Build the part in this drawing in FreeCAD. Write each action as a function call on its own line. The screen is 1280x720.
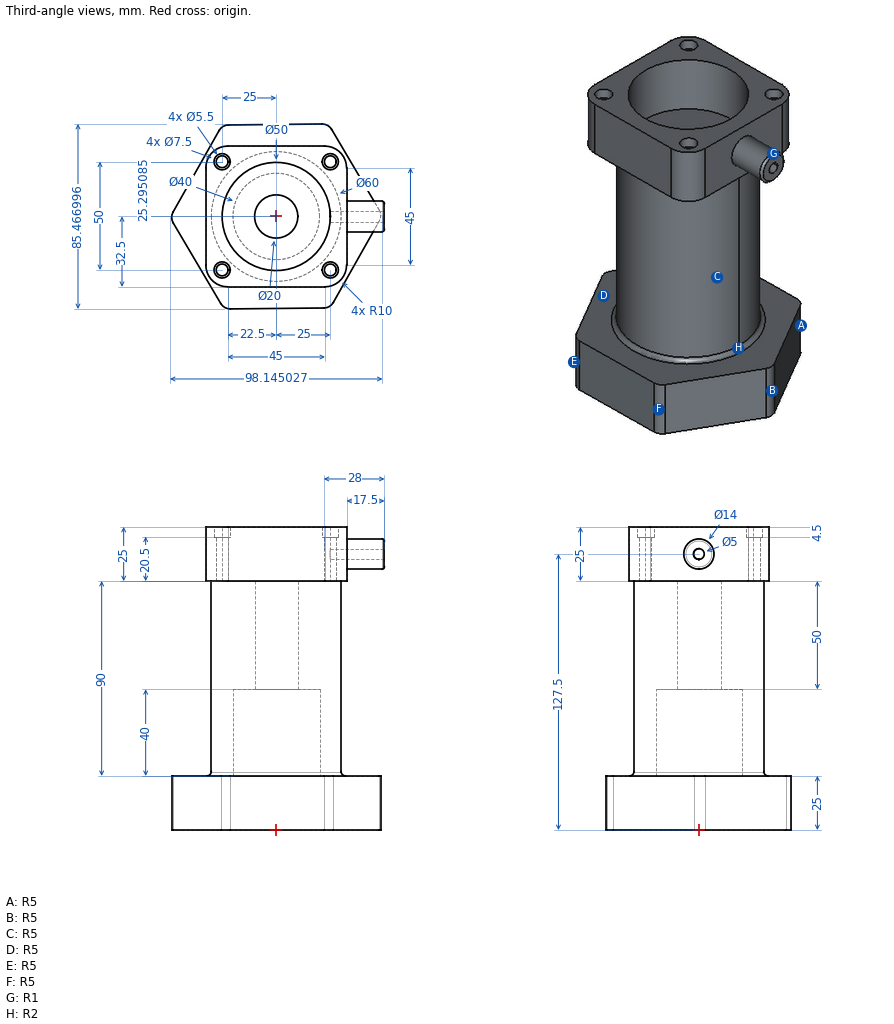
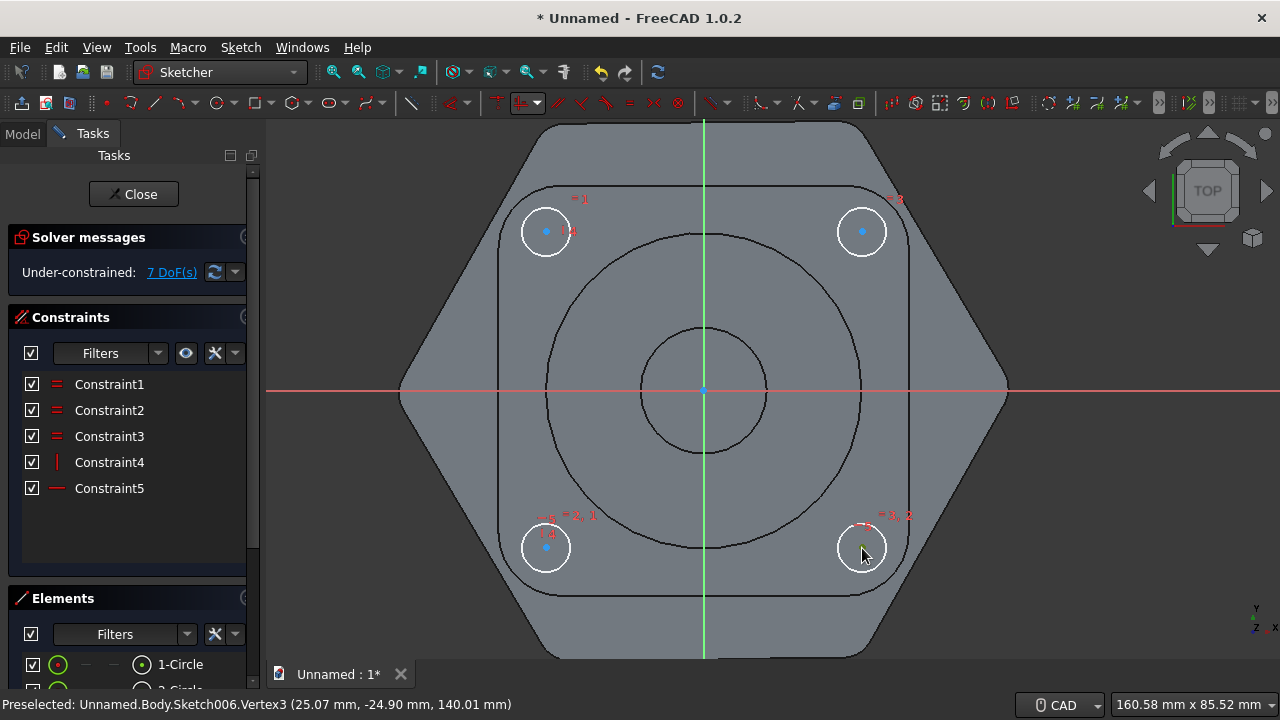
click(862, 232)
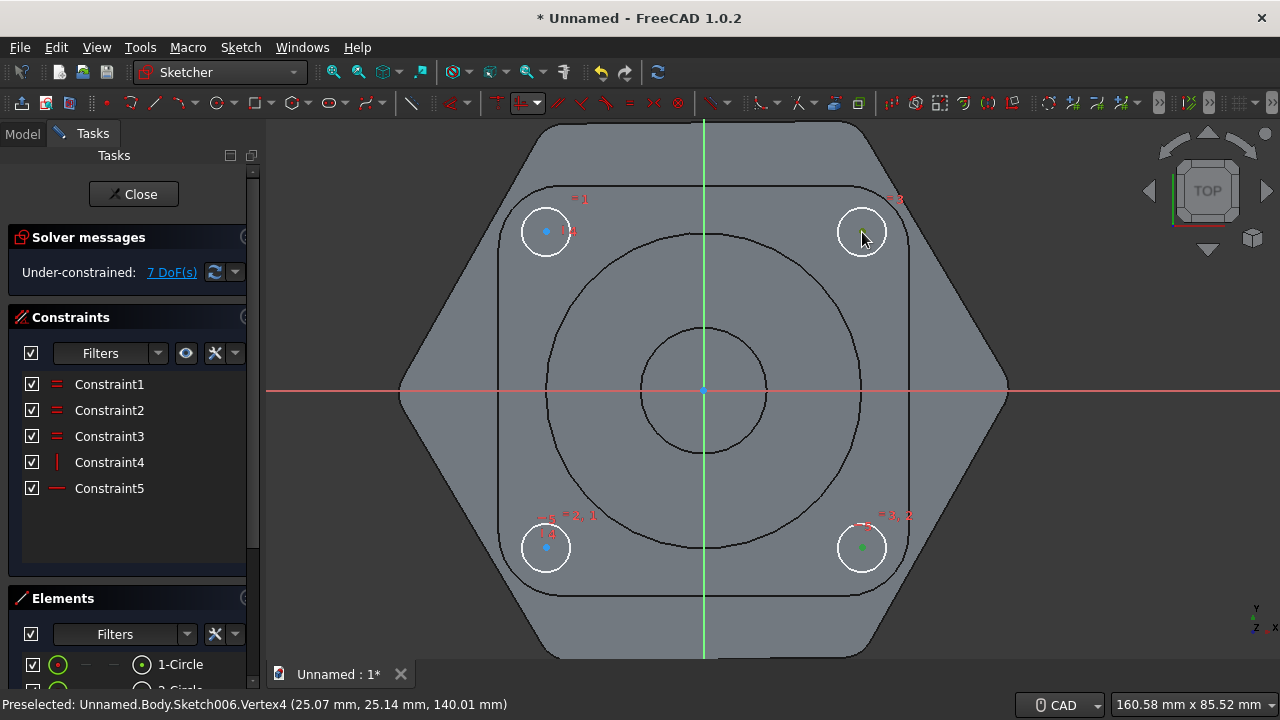
key(v)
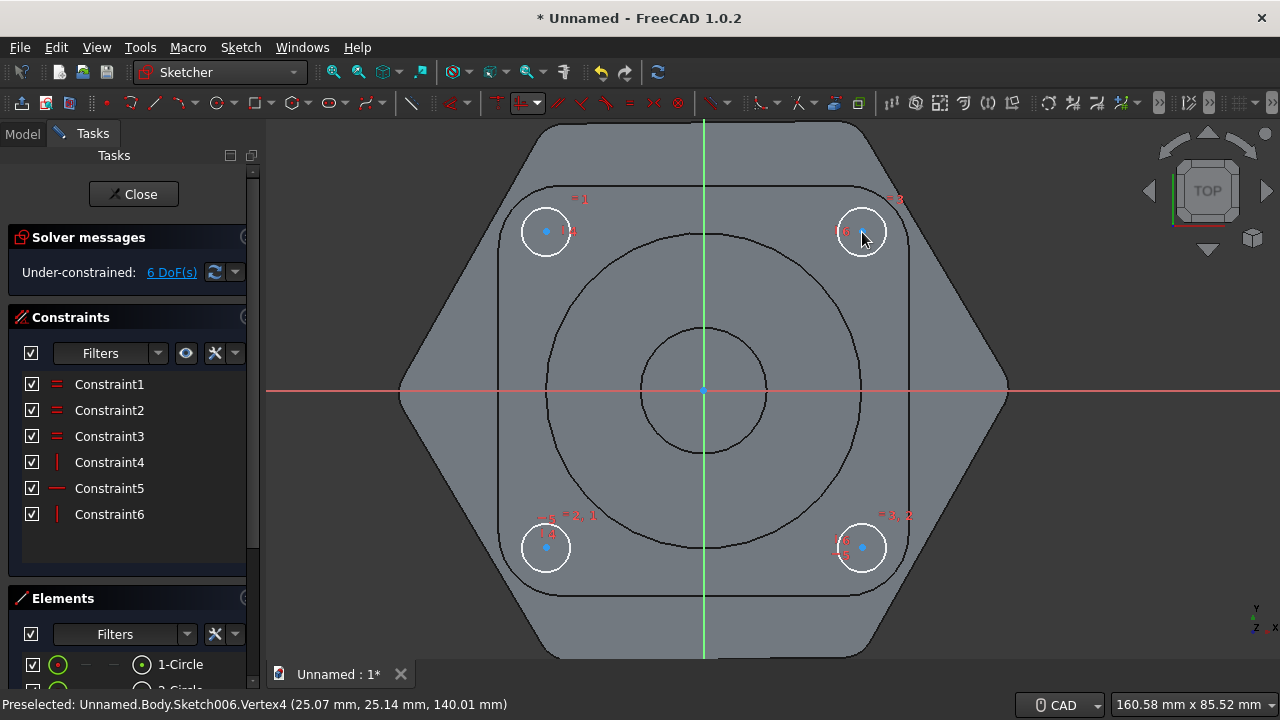
click(546, 232)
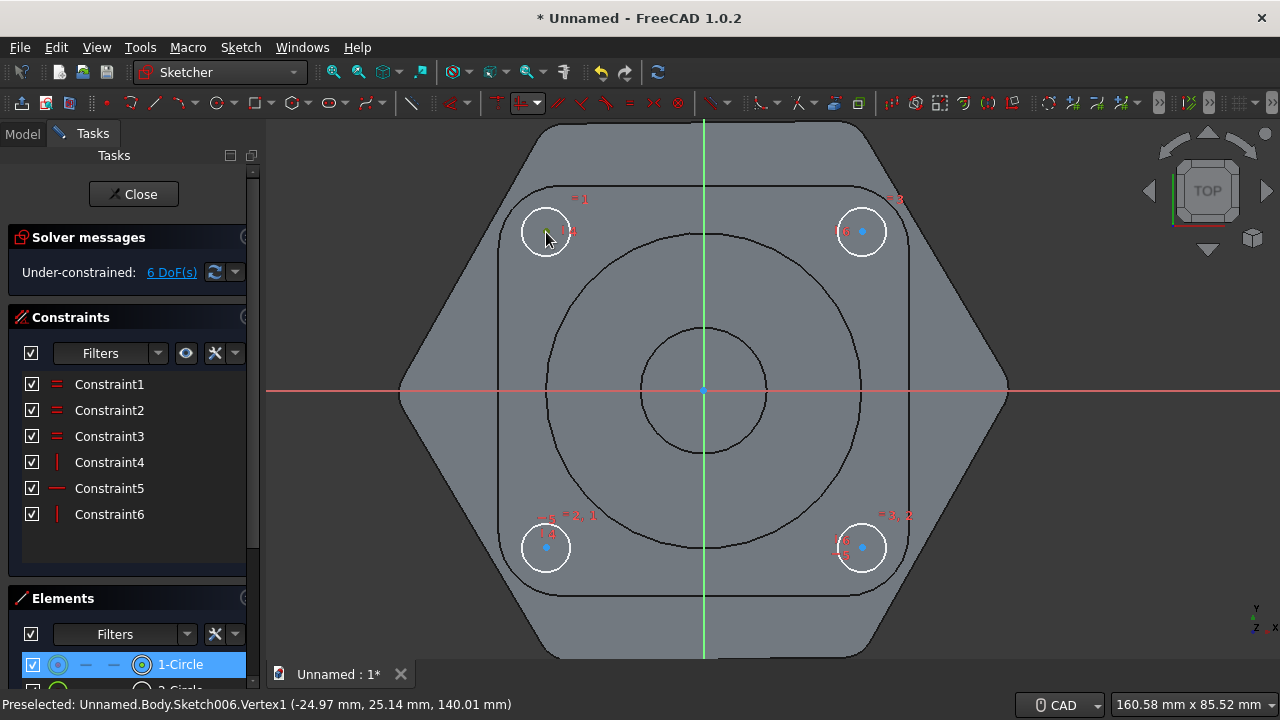
click(862, 232)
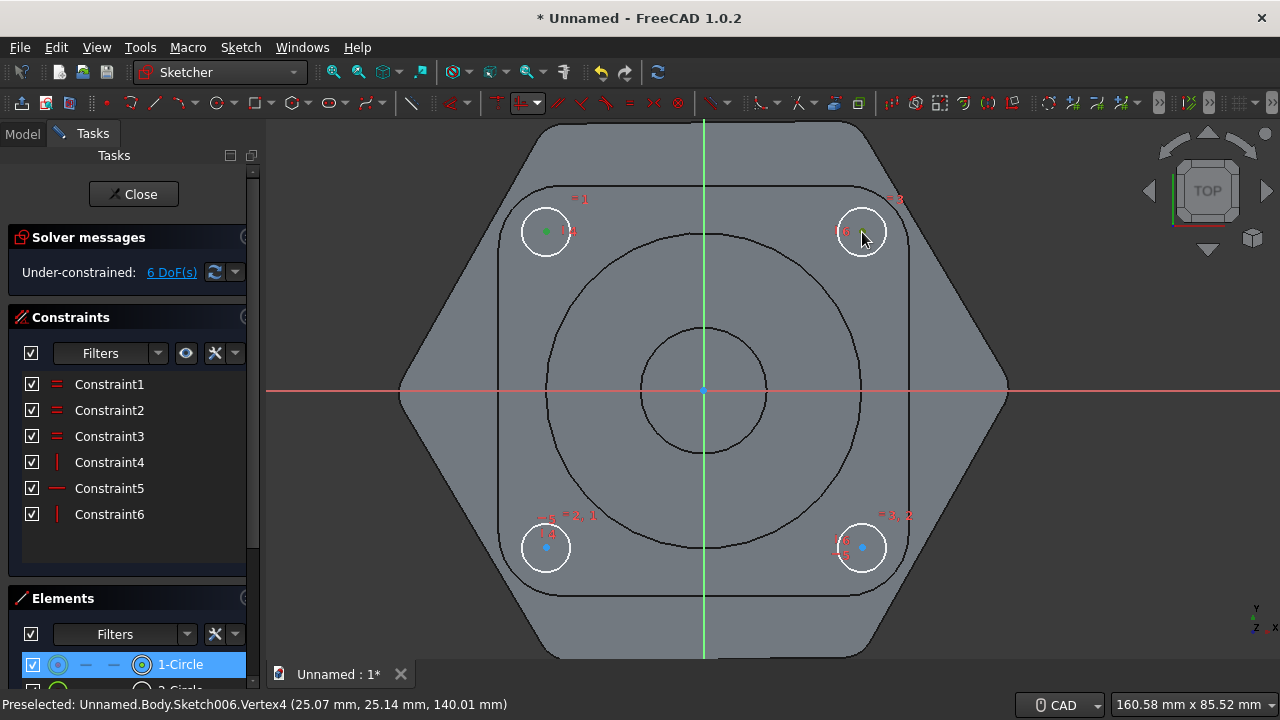
click(540, 104)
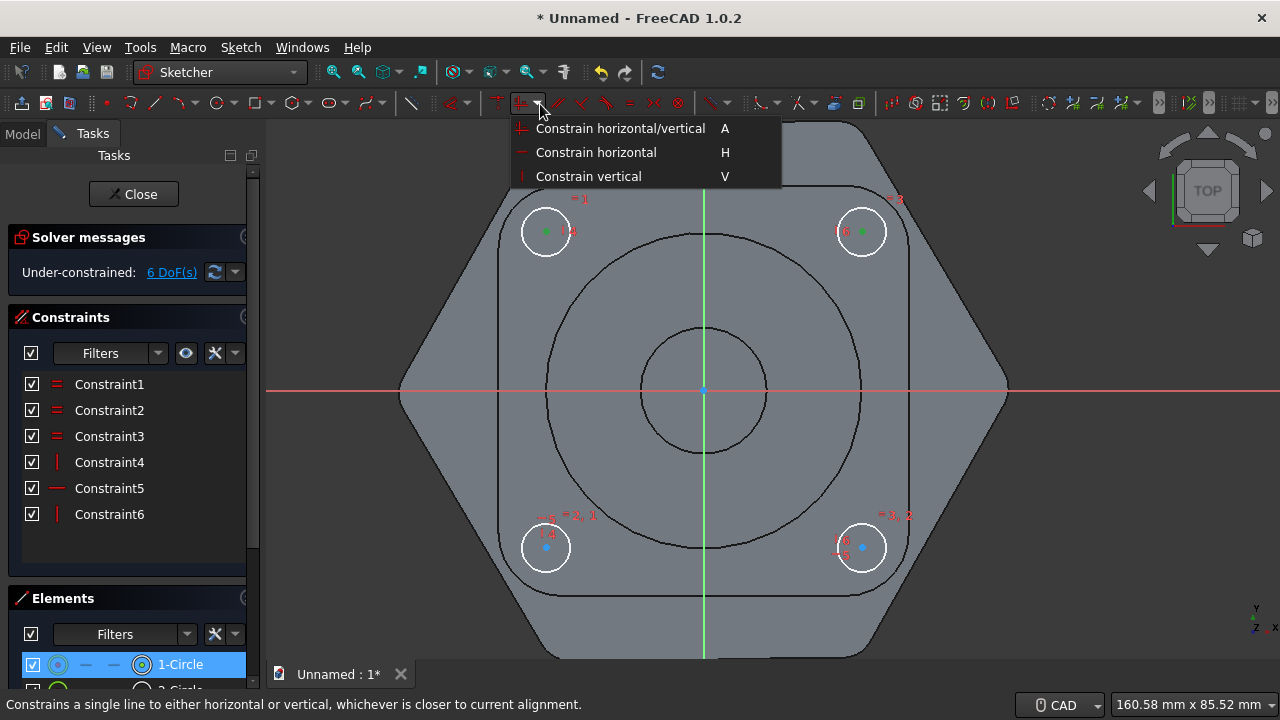
click(646, 152)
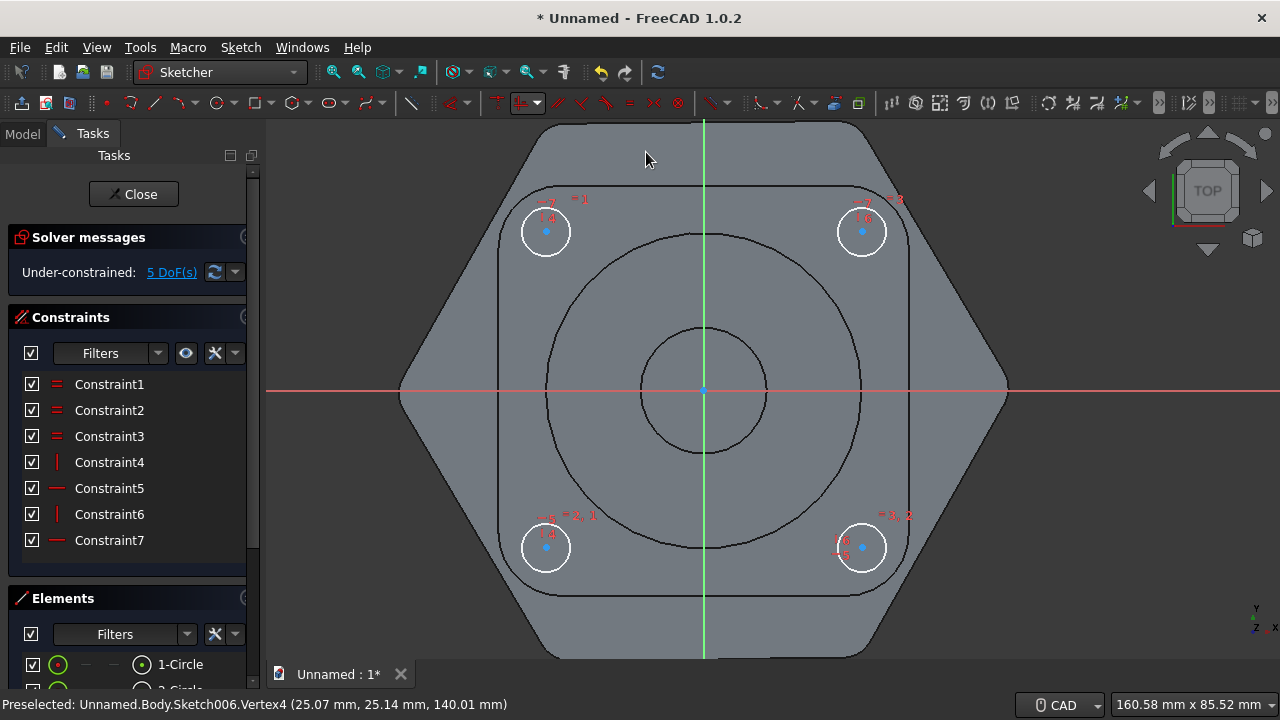
click(450, 104)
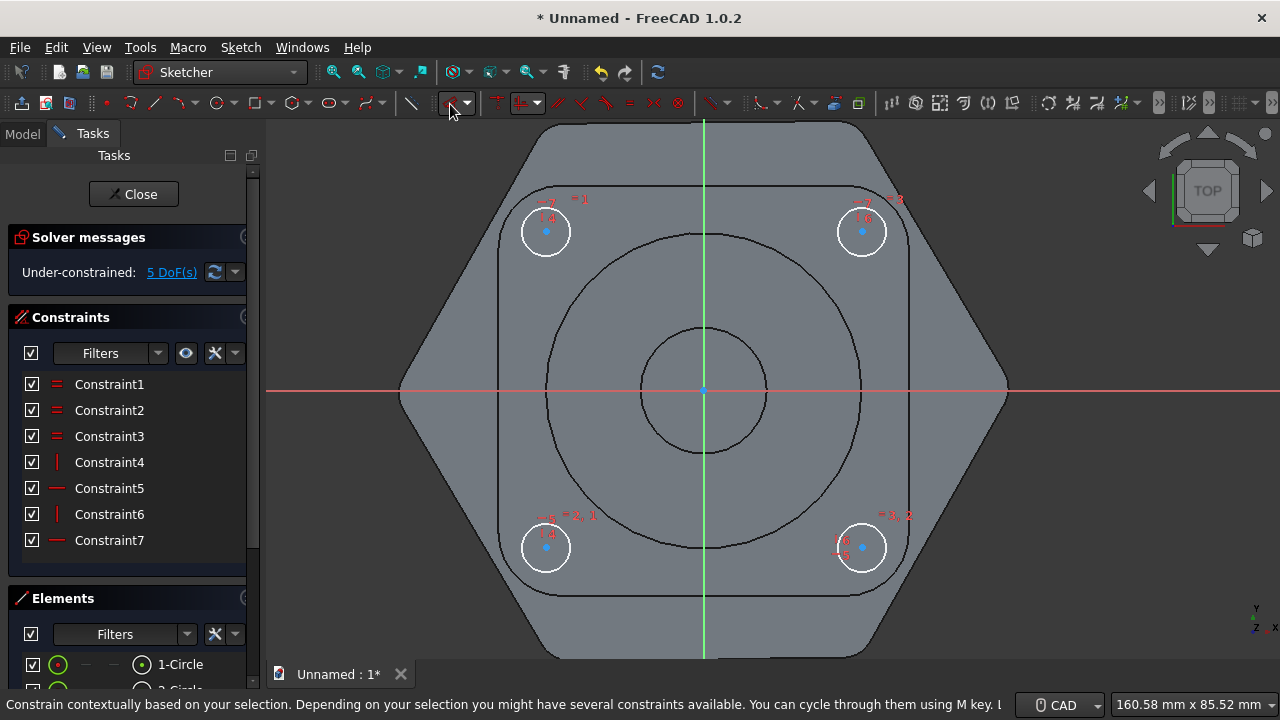
click(563, 215)
click(586, 192)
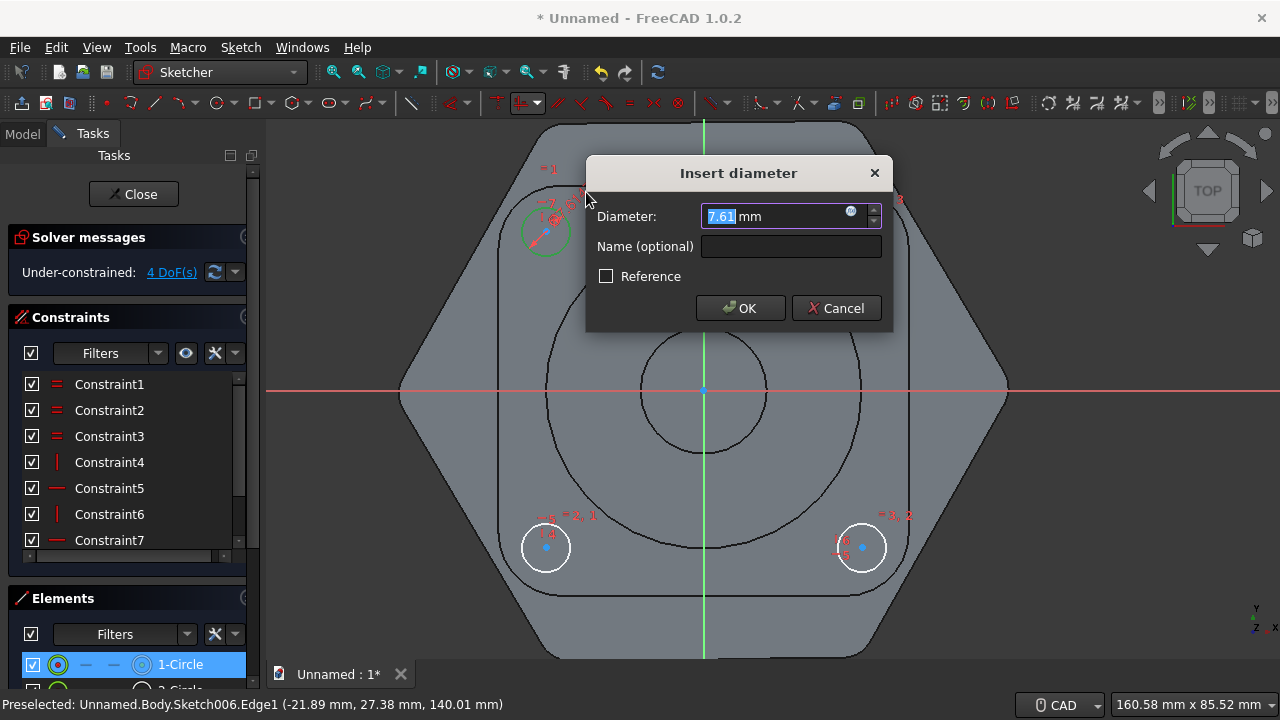
text(7.5)
key(Return)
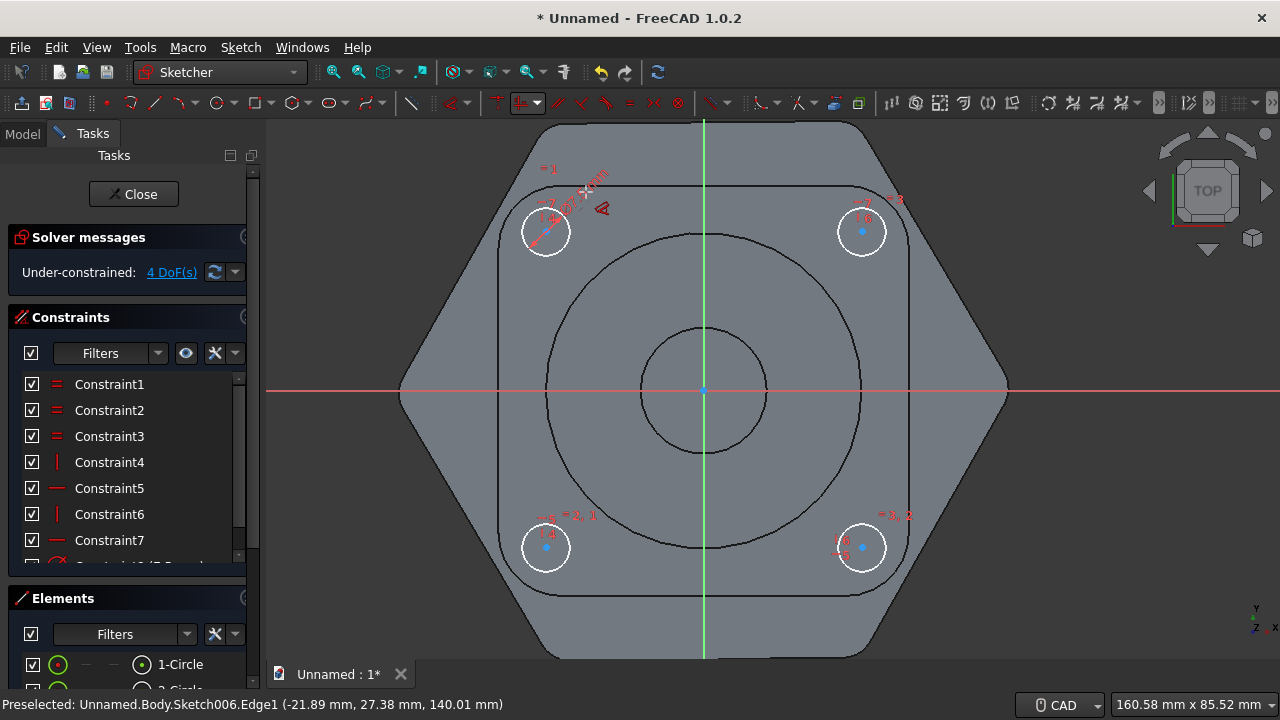
click(546, 232)
click(661, 198)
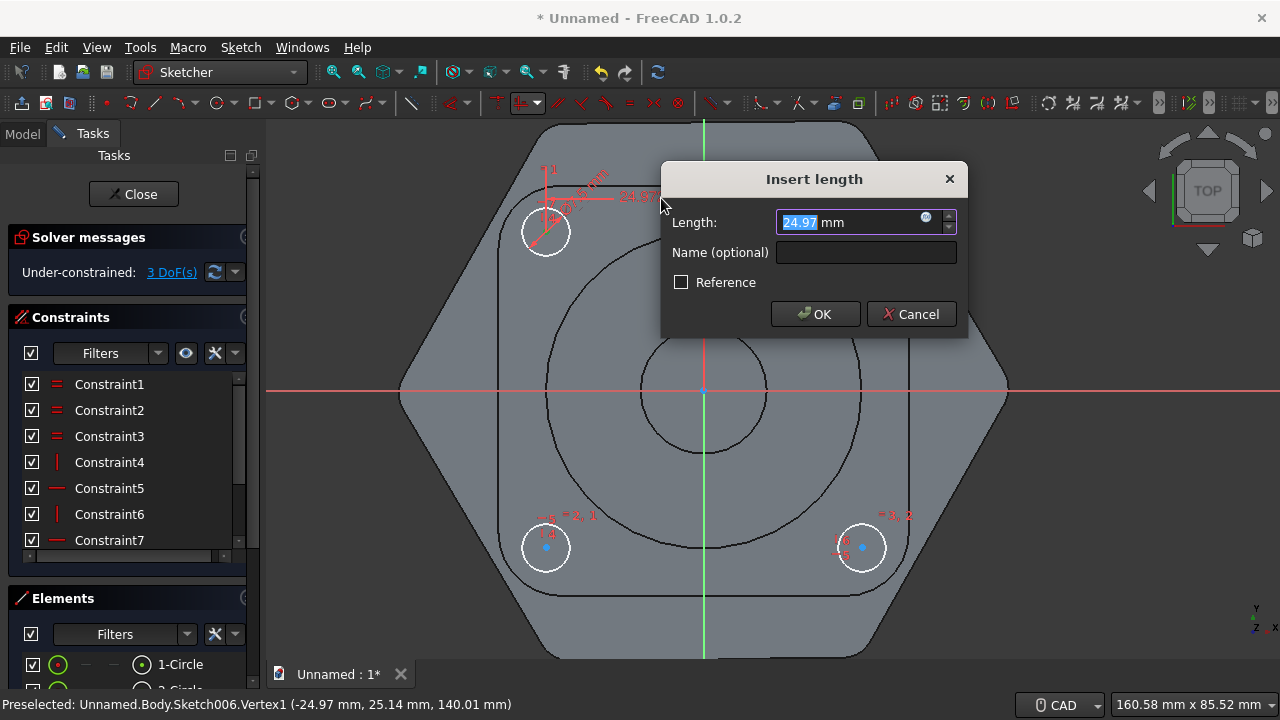
text(25)
key(Return)